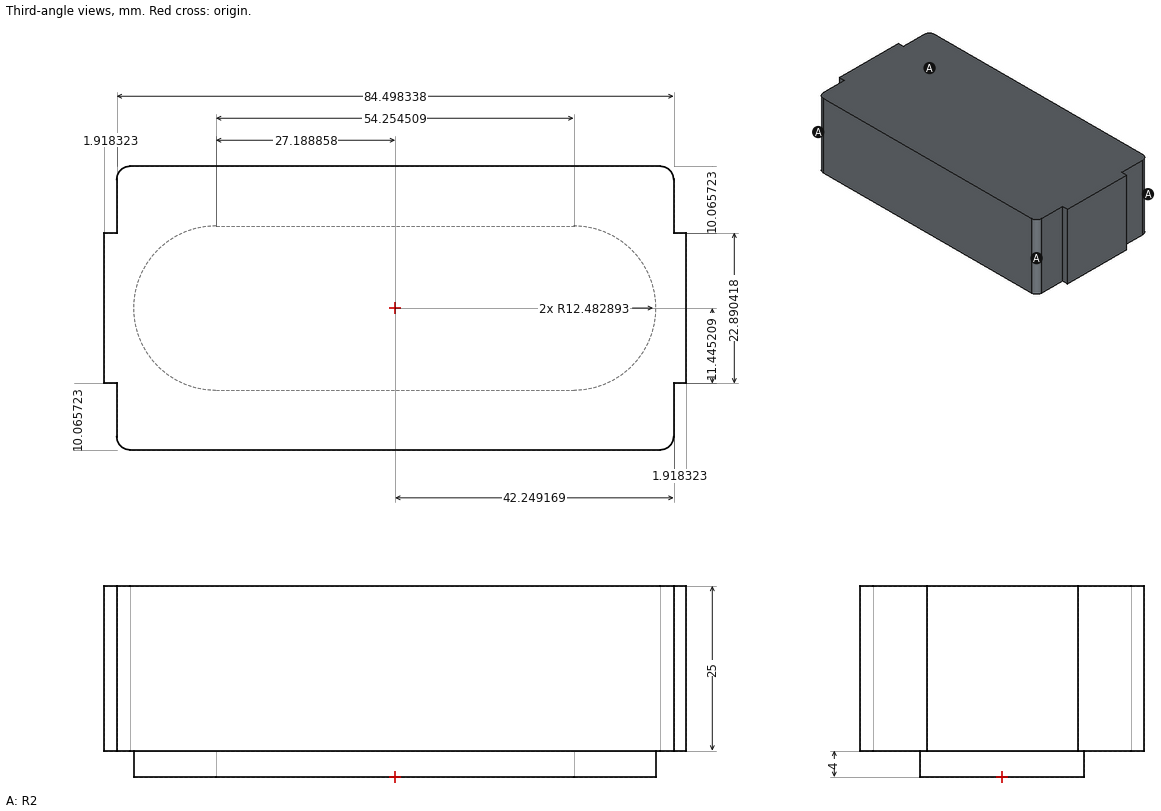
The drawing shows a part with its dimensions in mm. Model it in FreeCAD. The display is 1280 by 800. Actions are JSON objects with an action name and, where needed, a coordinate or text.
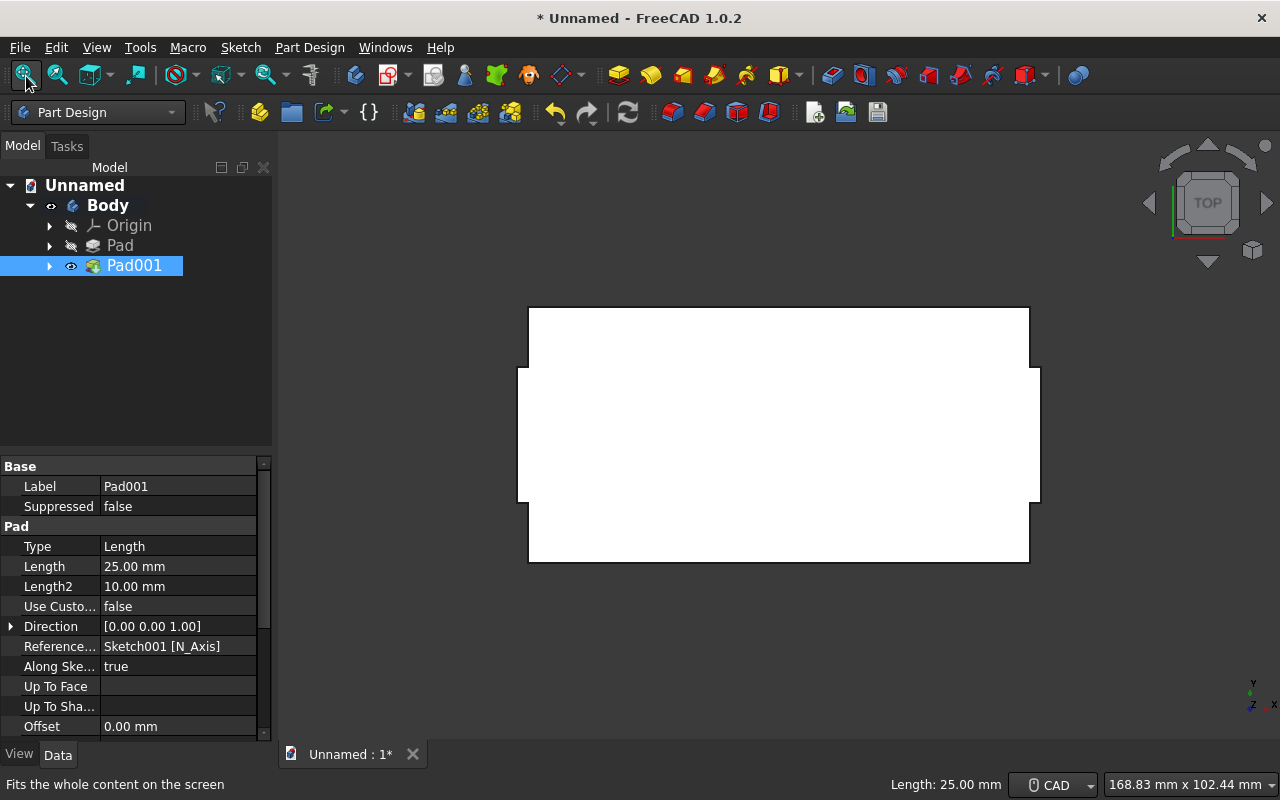
{"action": "key", "text": "1"}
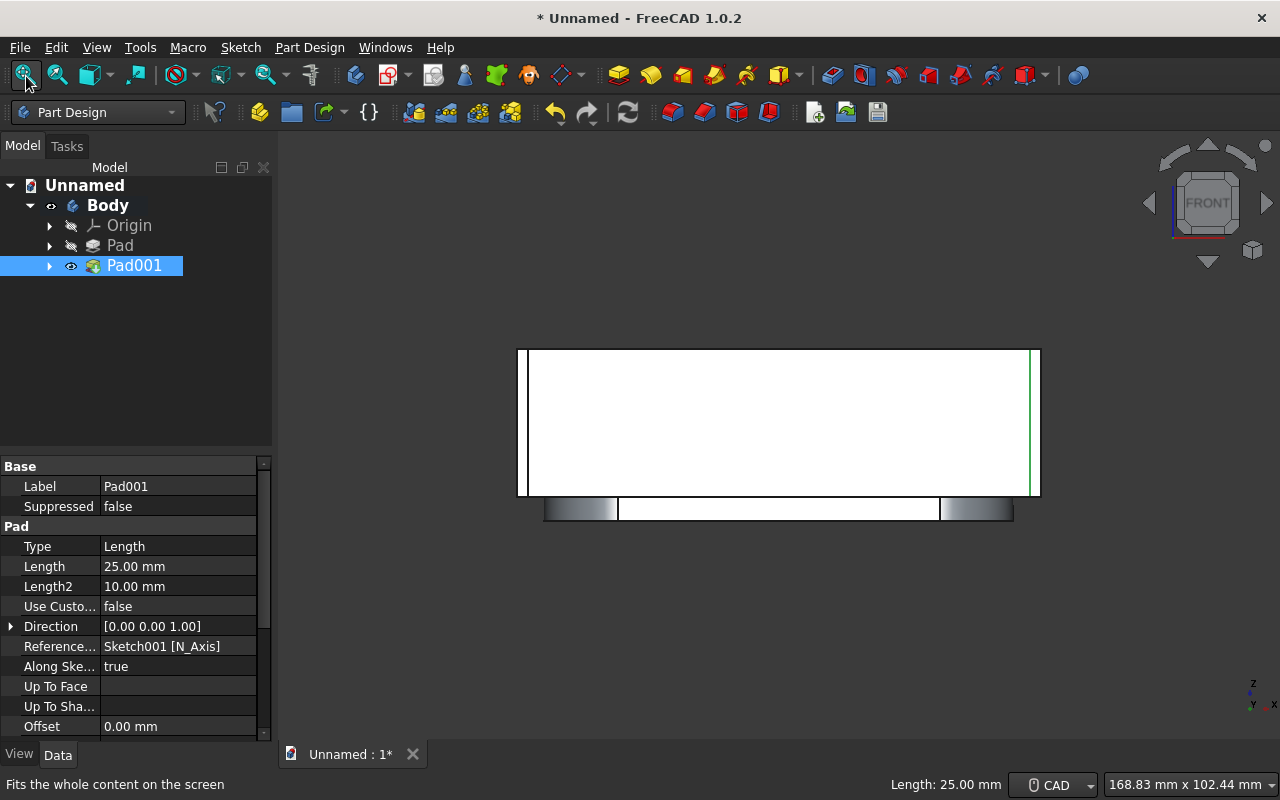
{"action": "left_click", "coordinate": [528, 422], "text": "ctrl"}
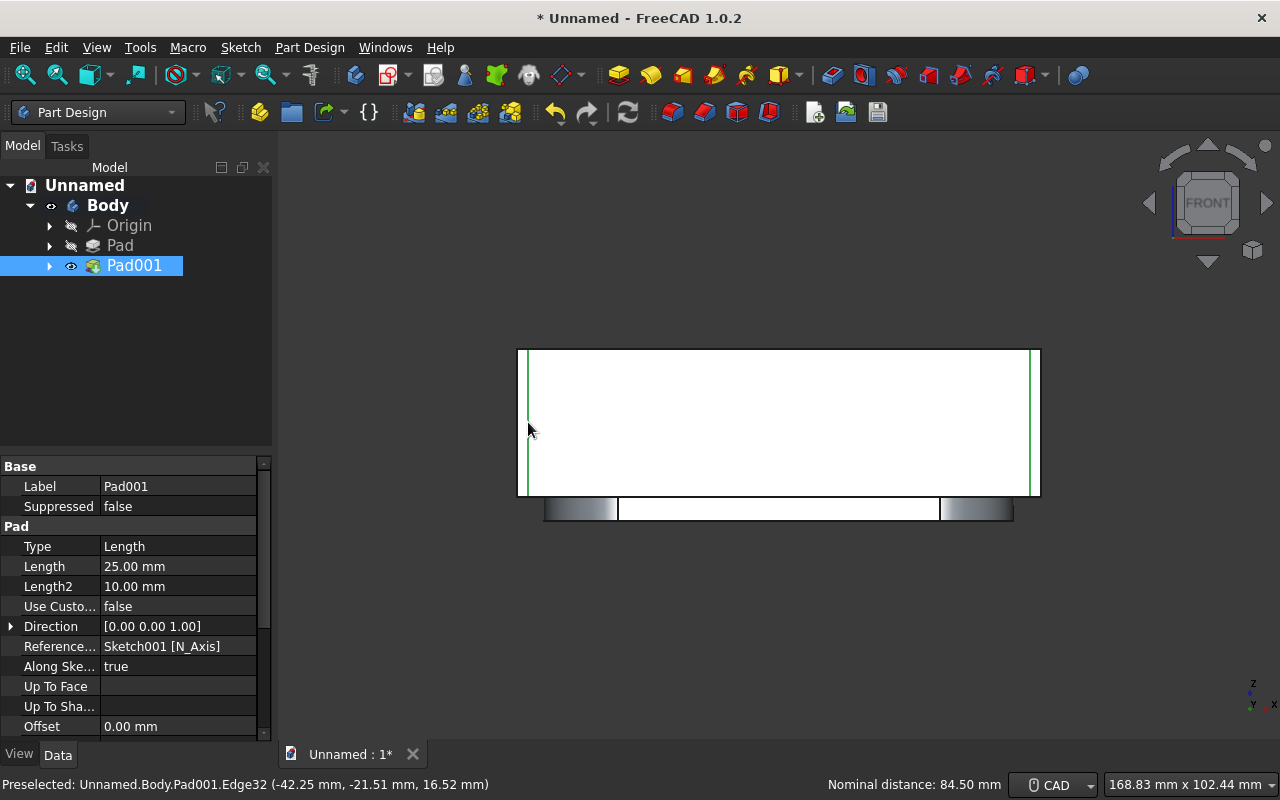
{"action": "key", "text": "3"}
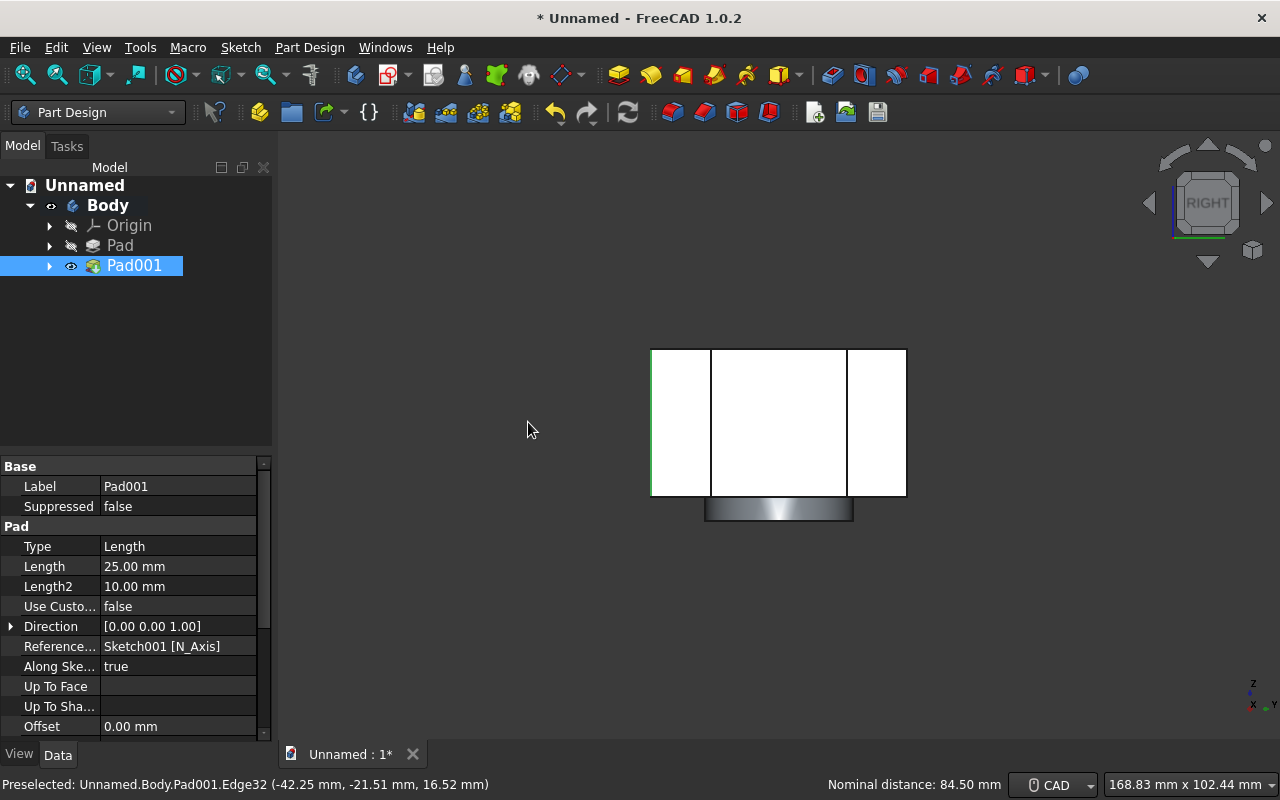
{"action": "left_click", "coordinate": [26, 76]}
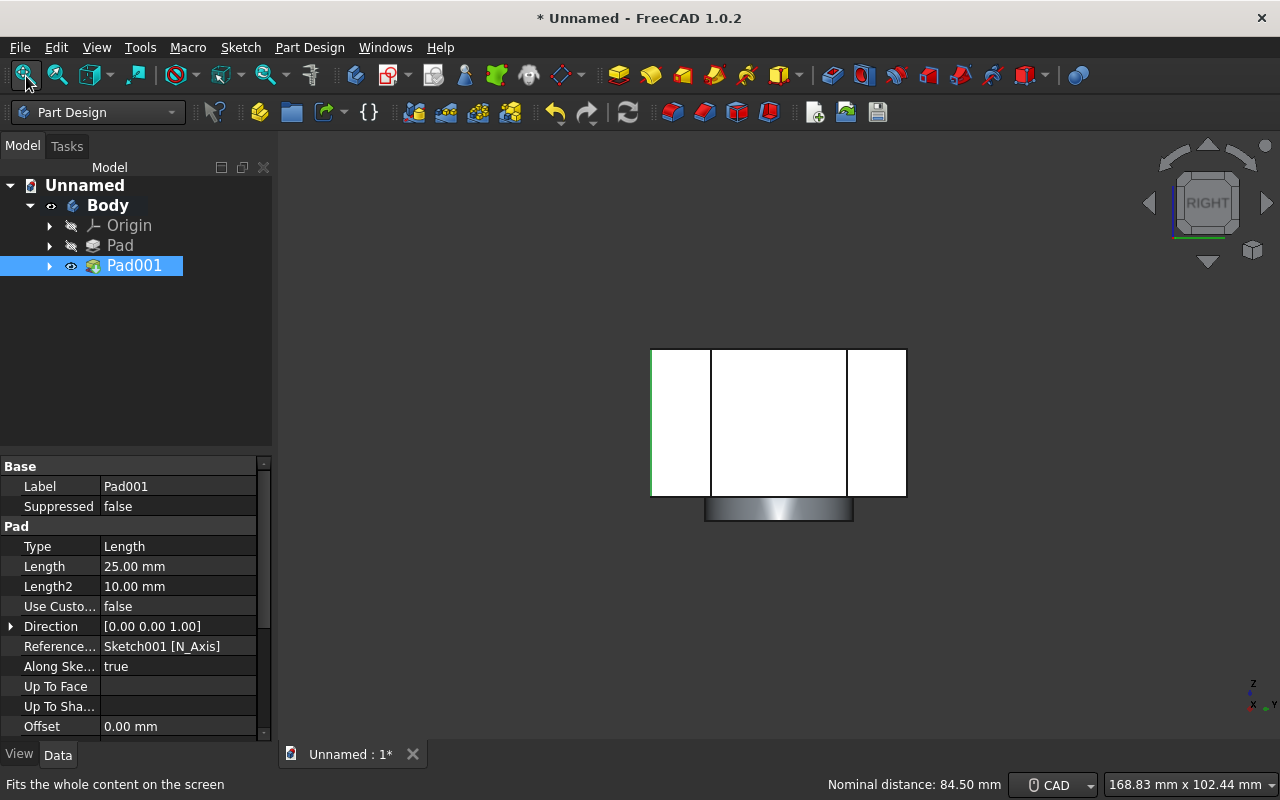
{"action": "left_click", "coordinate": [907, 422], "text": "ctrl"}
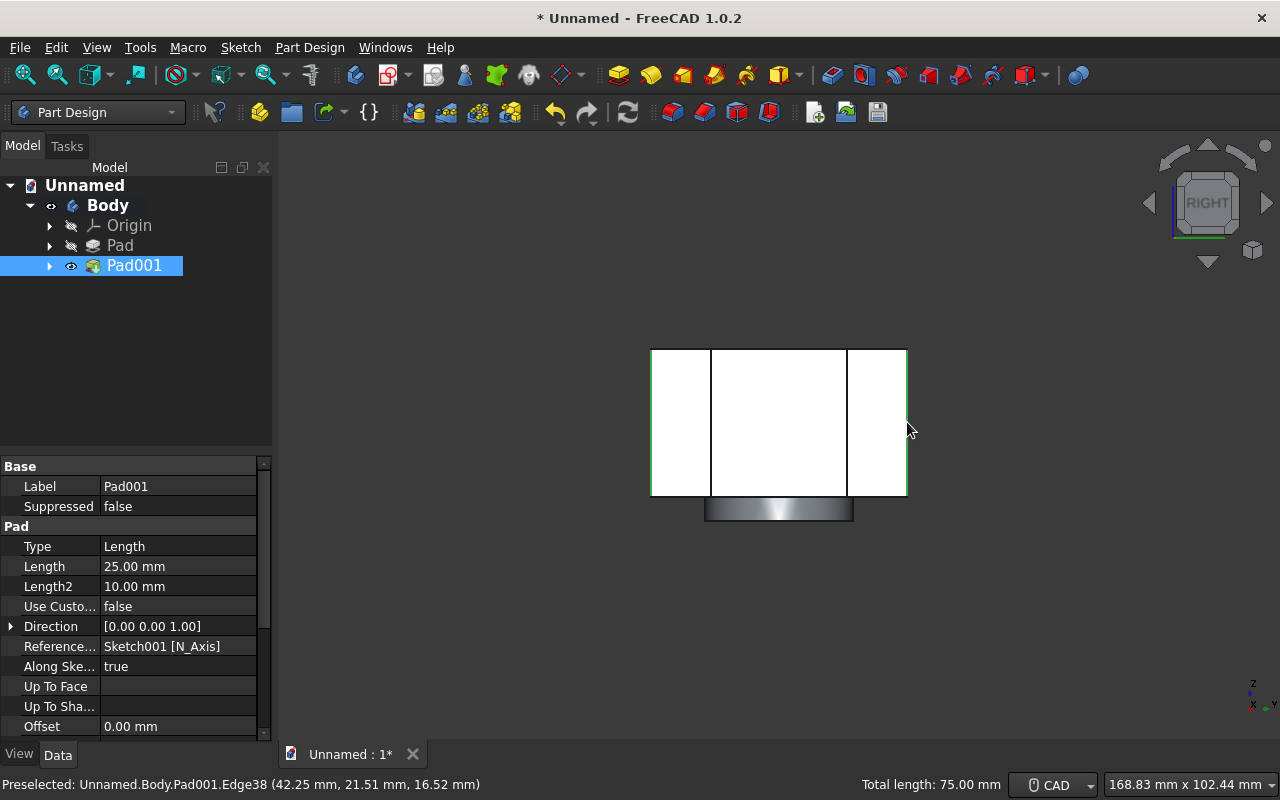
{"action": "key", "text": "5"}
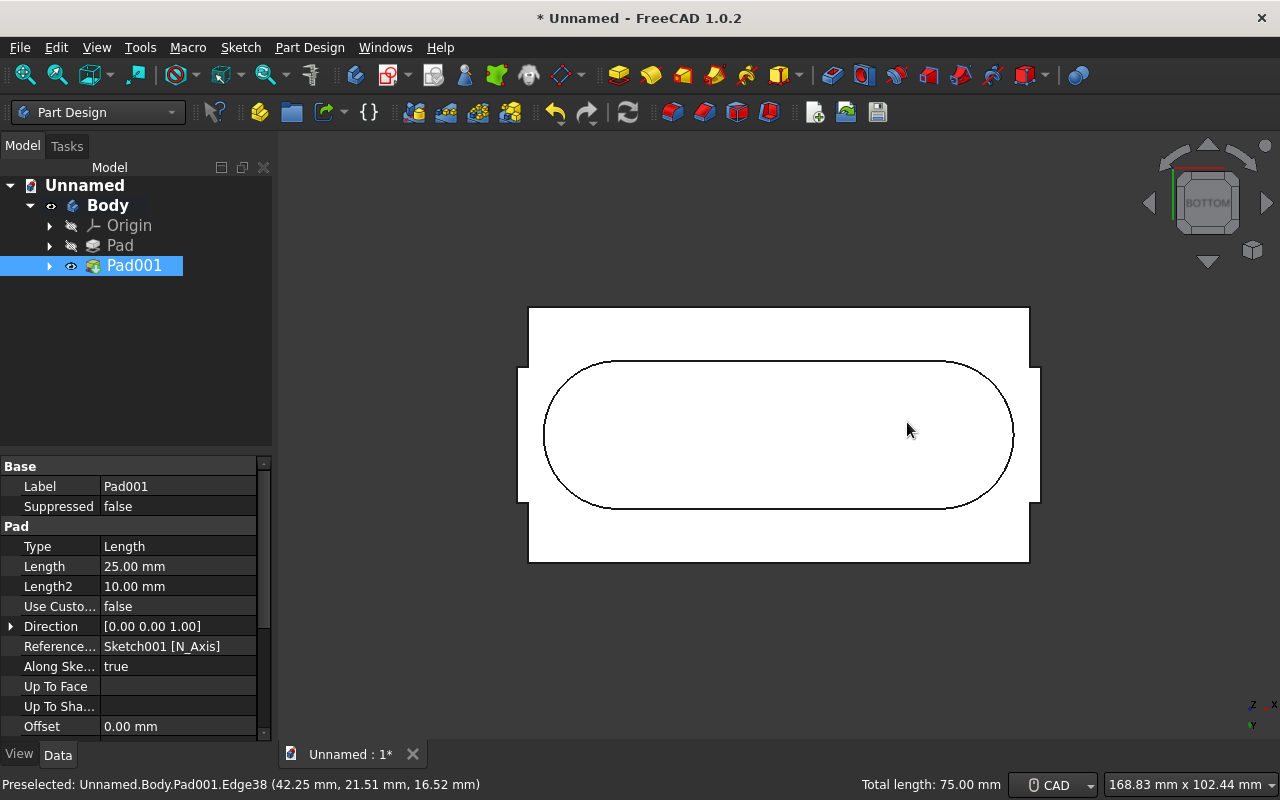
{"action": "key", "text": "4"}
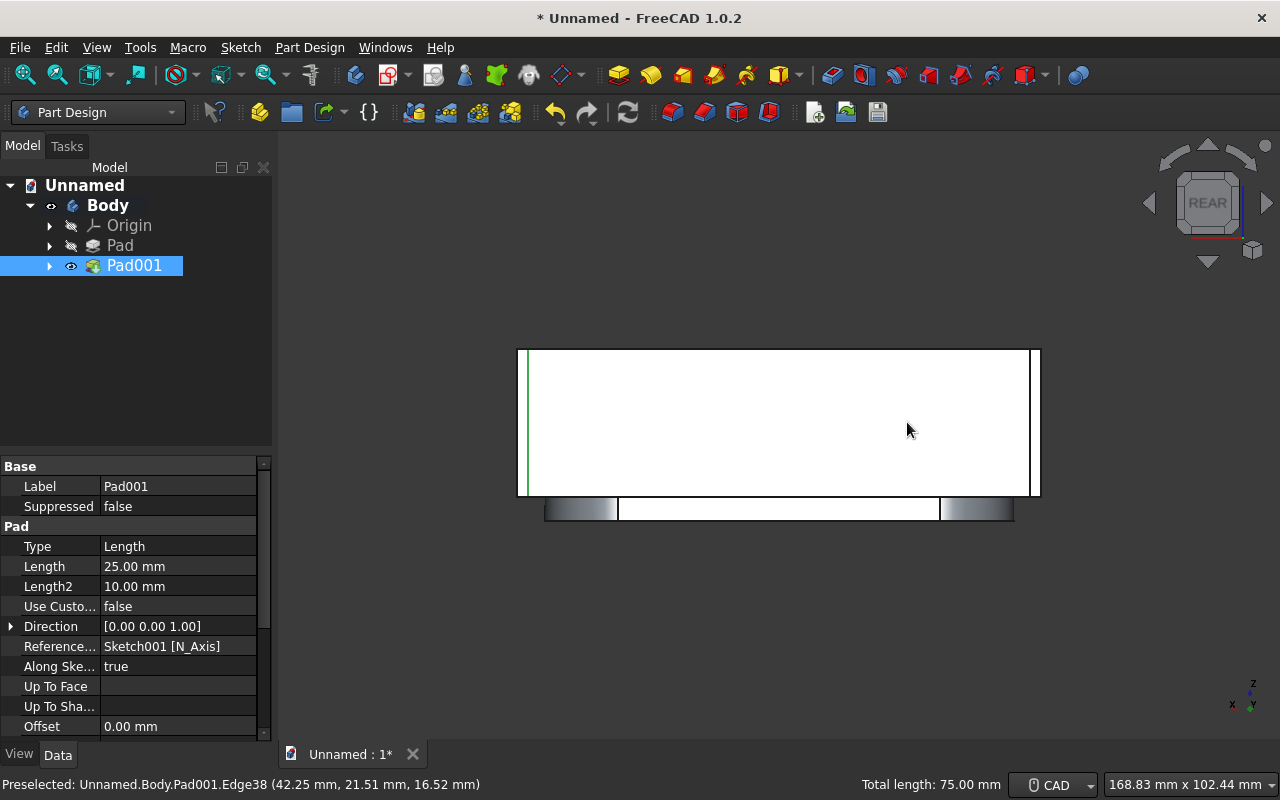
{"action": "left_click", "coordinate": [1030, 422], "text": "ctrl"}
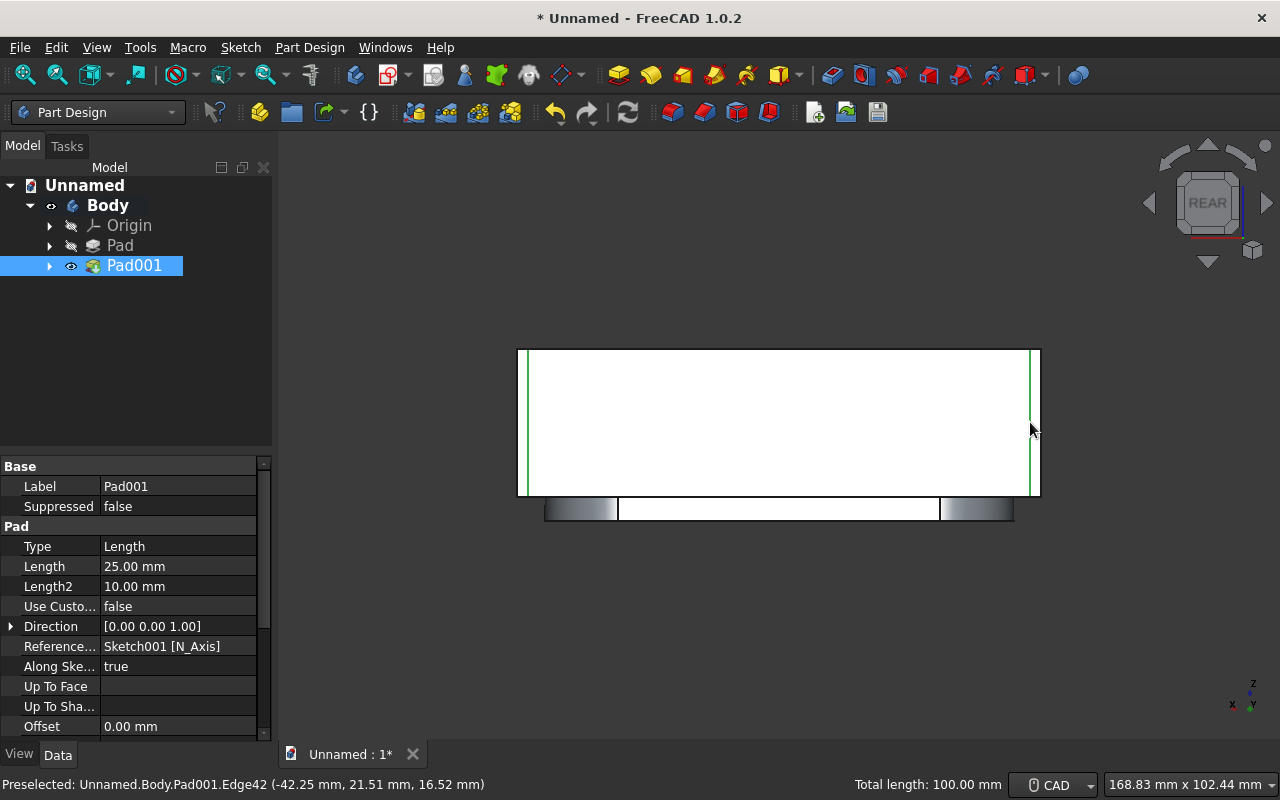
{"action": "left_click", "coordinate": [674, 112]}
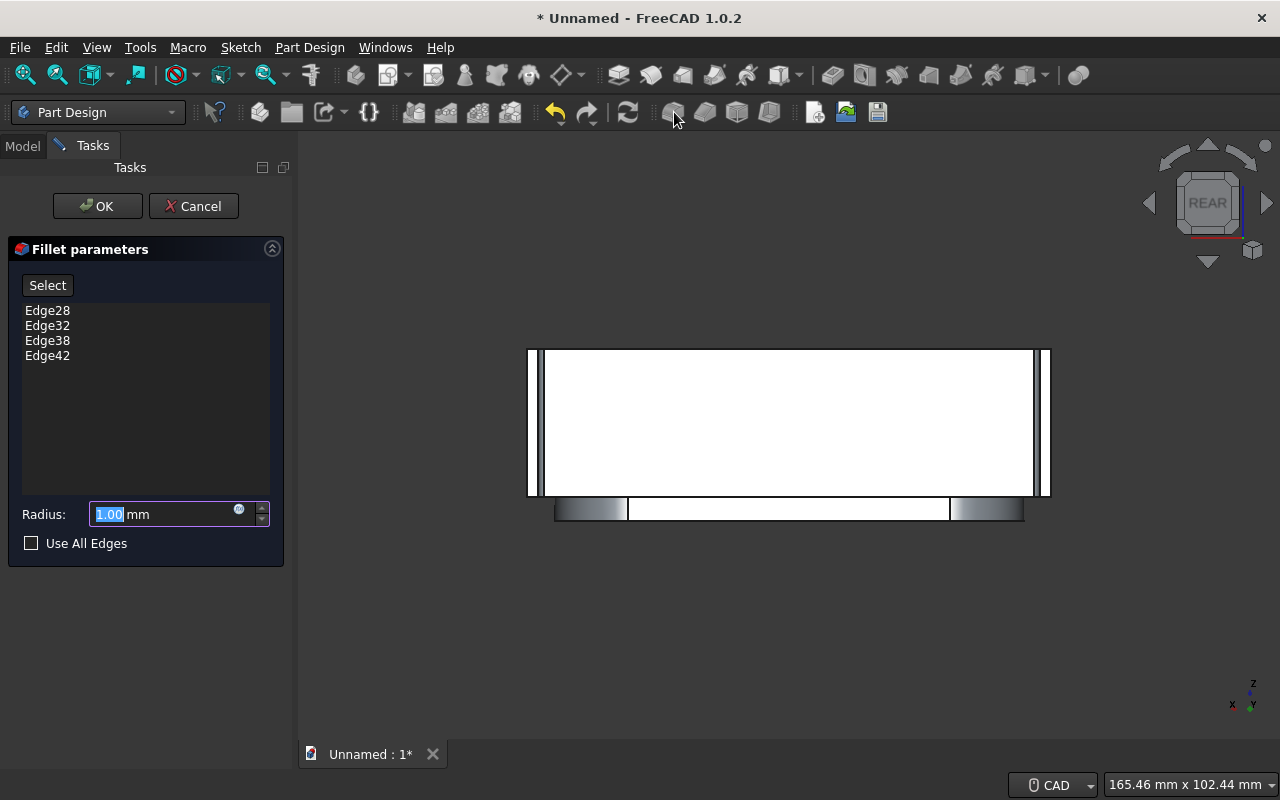
{"action": "type", "text": "2"}
{"action": "key", "text": "Tab"}